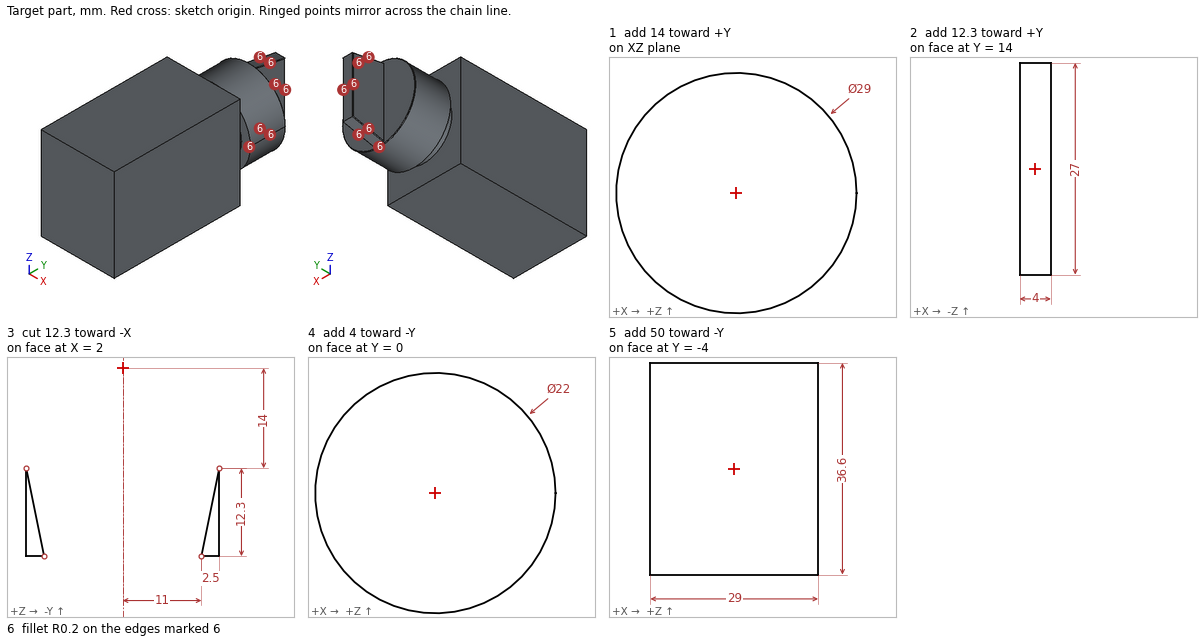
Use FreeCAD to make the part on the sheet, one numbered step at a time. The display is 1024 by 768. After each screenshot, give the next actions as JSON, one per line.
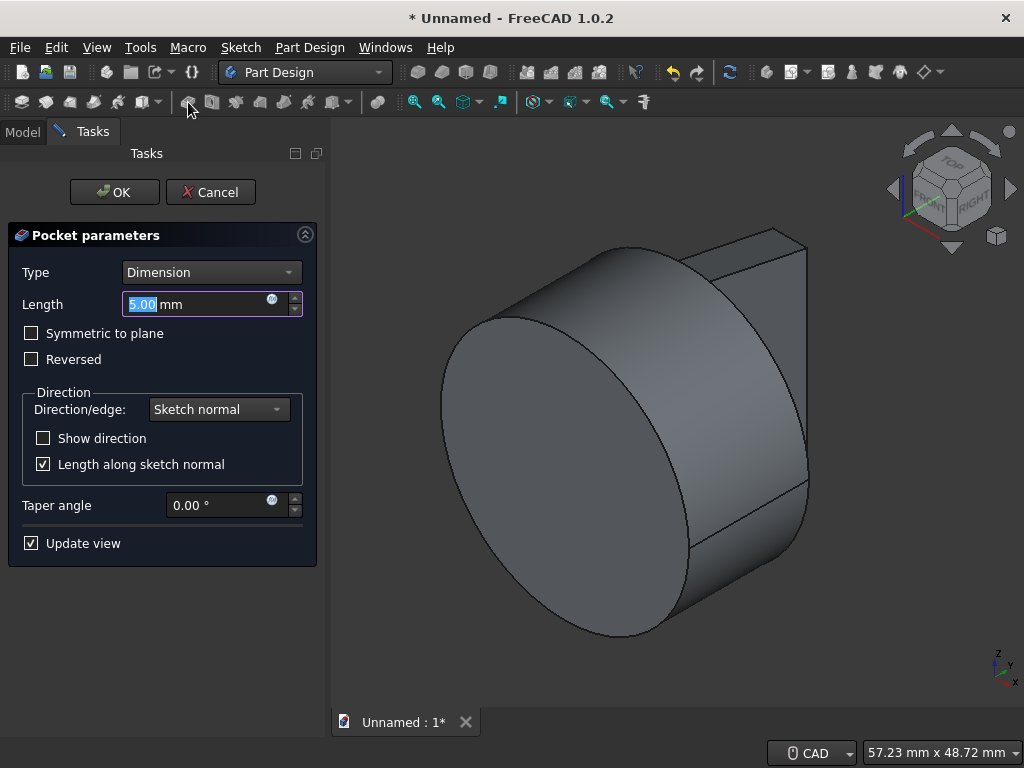
{"action": "type", "text": "12.3"}
{"action": "key", "text": "Tab"}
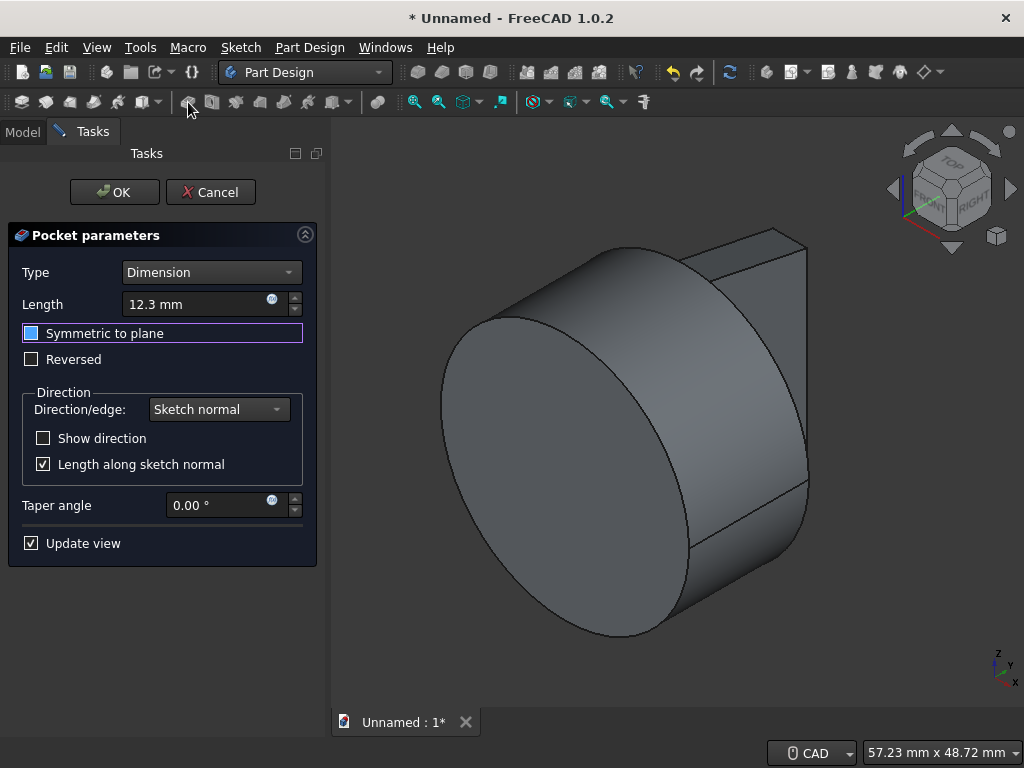
{"action": "left_click", "coordinate": [115, 192]}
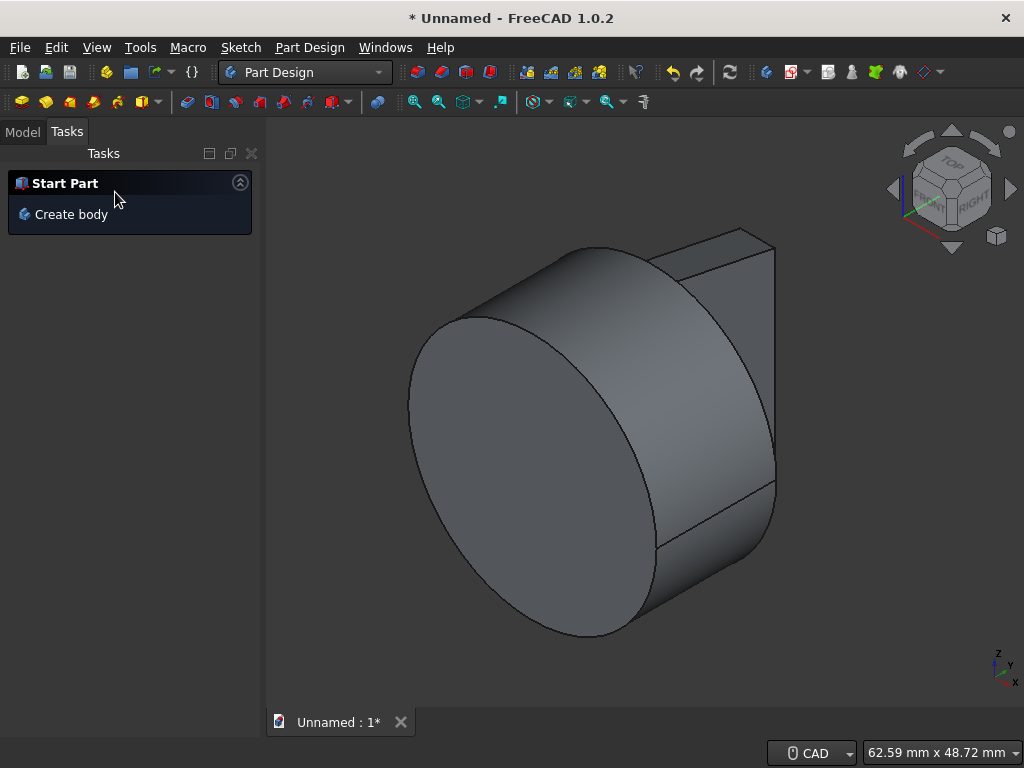
{"action": "left_click", "coordinate": [532, 476]}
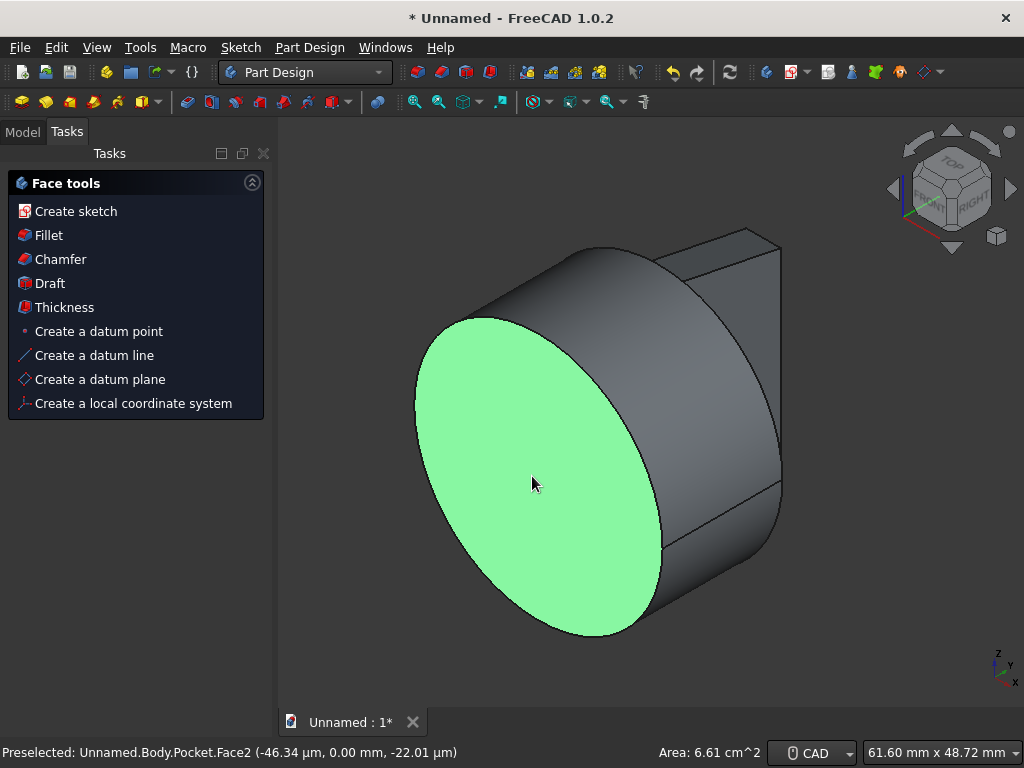
{"action": "left_click", "coordinate": [792, 72]}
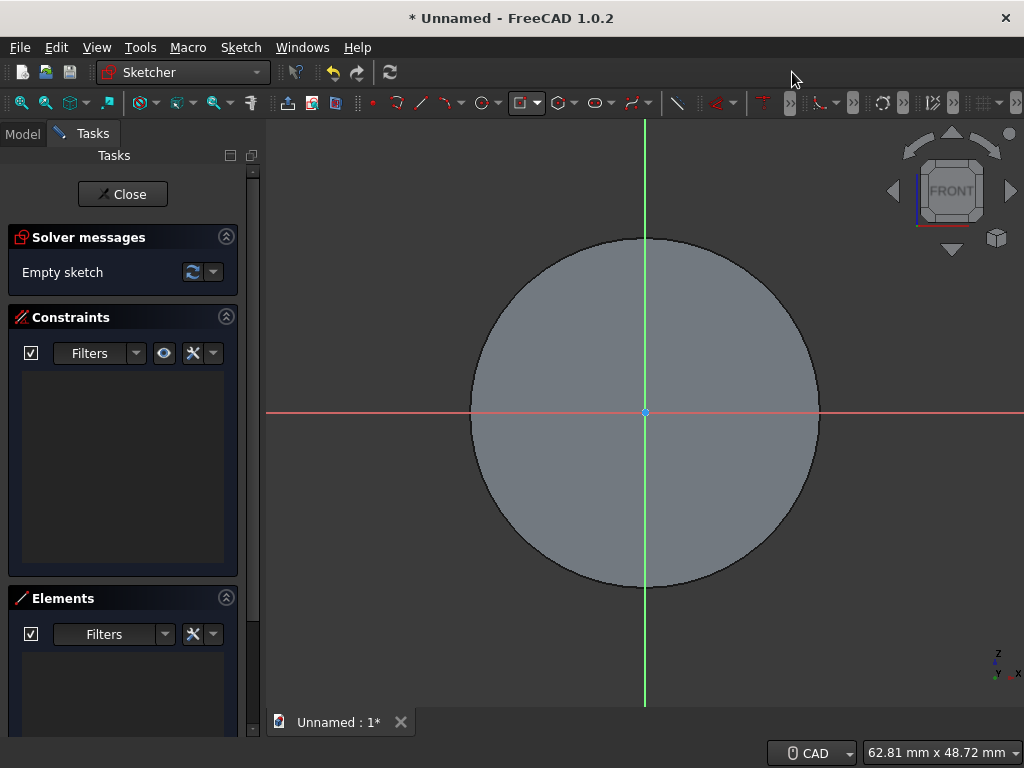
{"action": "scroll", "coordinate": [784, 413], "scroll_direction": "up", "scroll_amount": 2}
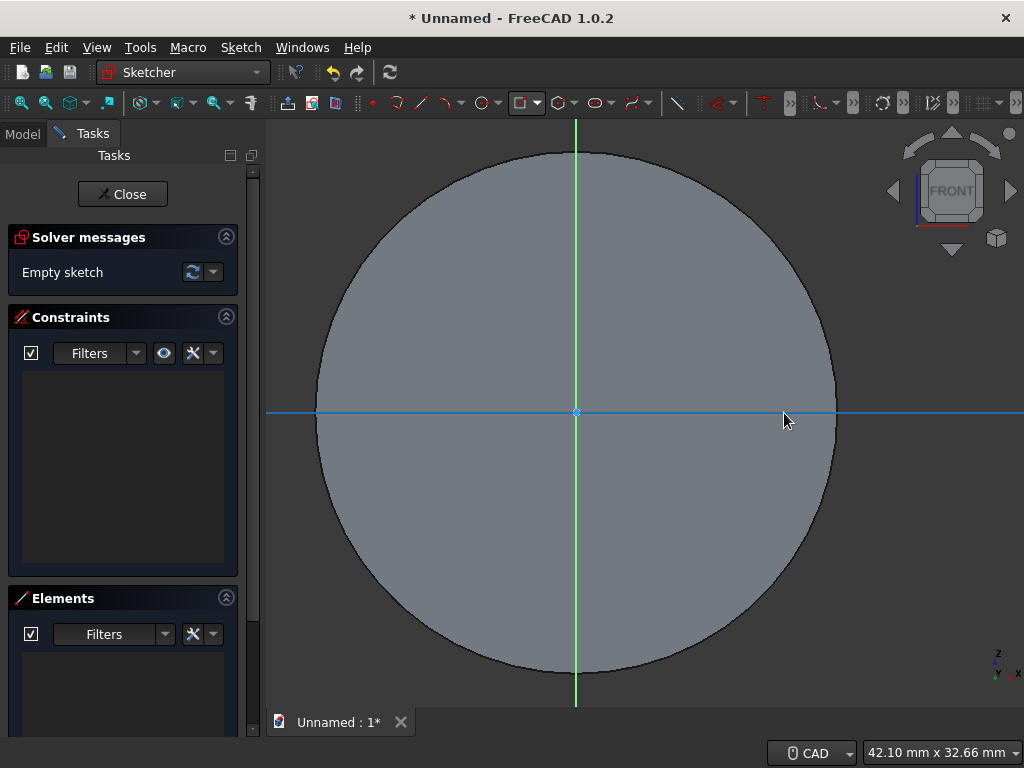
{"action": "left_click", "coordinate": [482, 104]}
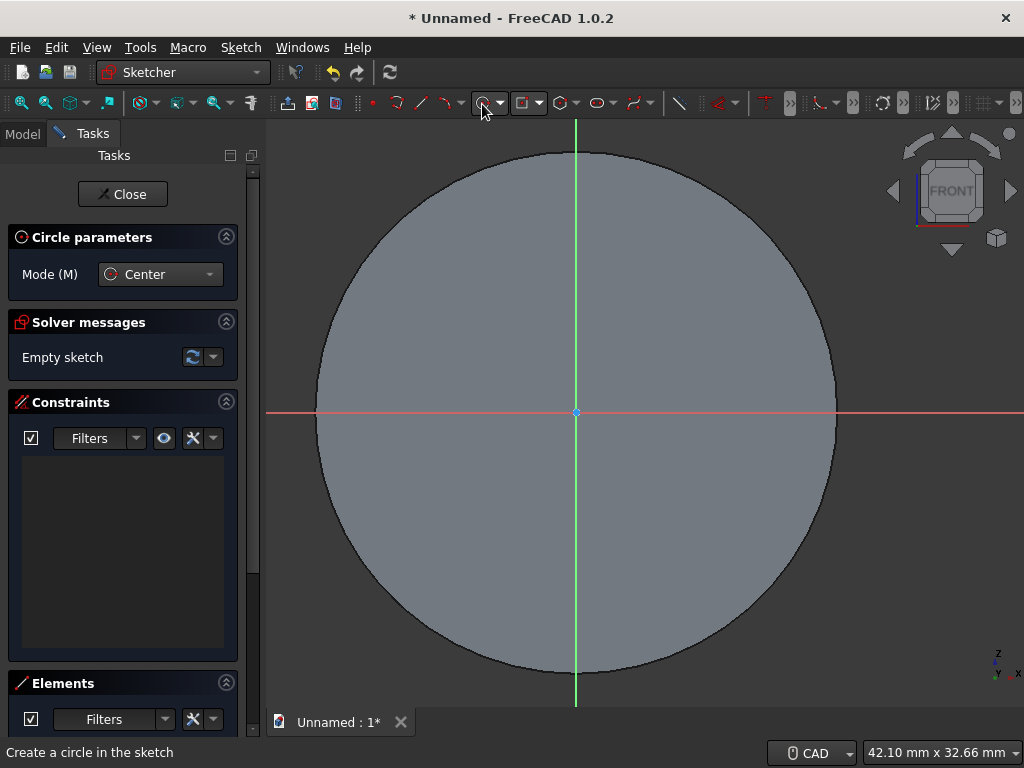
{"action": "left_click", "coordinate": [576, 413]}
{"action": "mouse_move", "coordinate": [716, 273]}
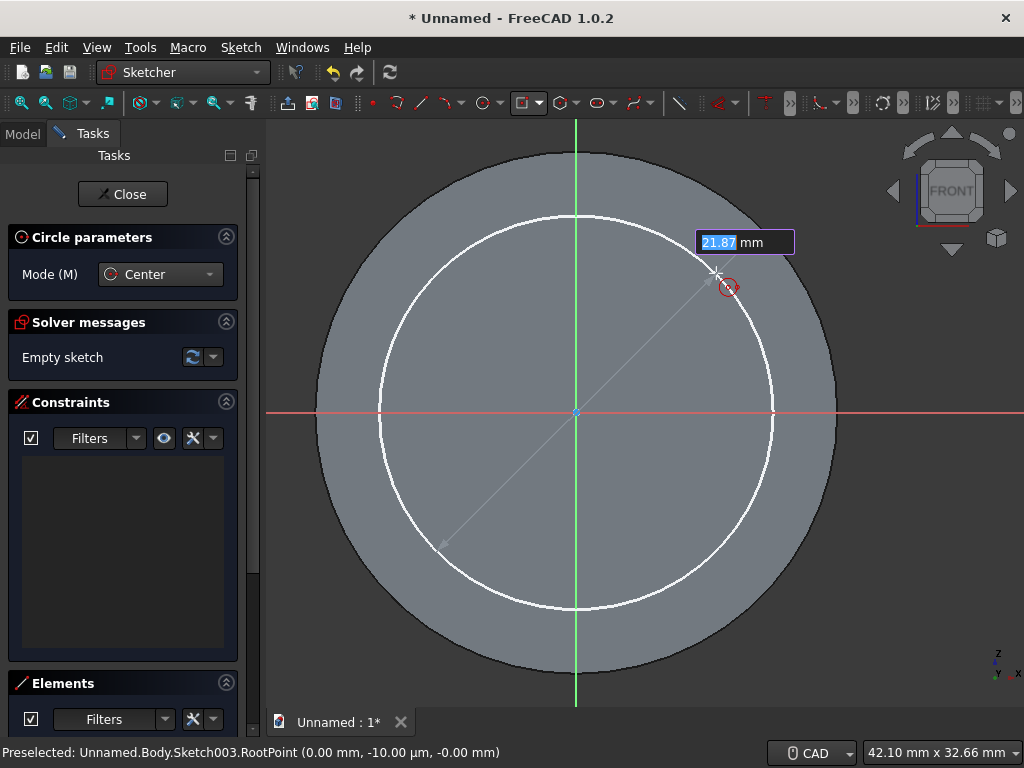
{"action": "type", "text": "22"}
{"action": "key", "text": "Return"}
{"action": "key", "text": "Escape"}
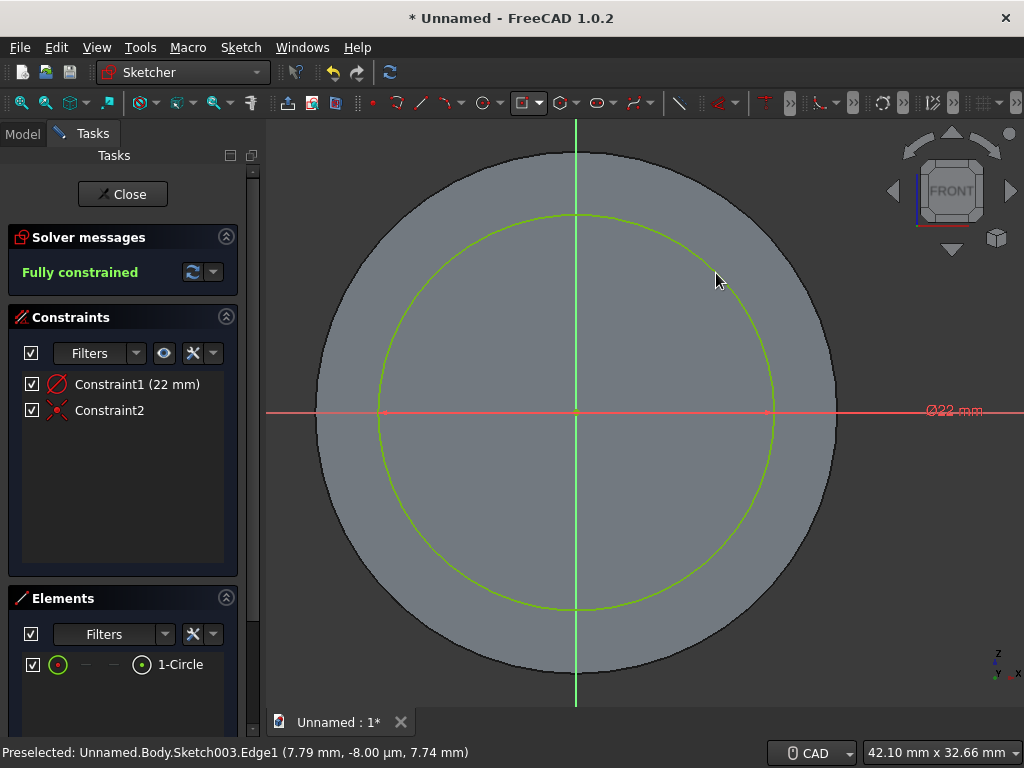
{"action": "left_click", "coordinate": [123, 194]}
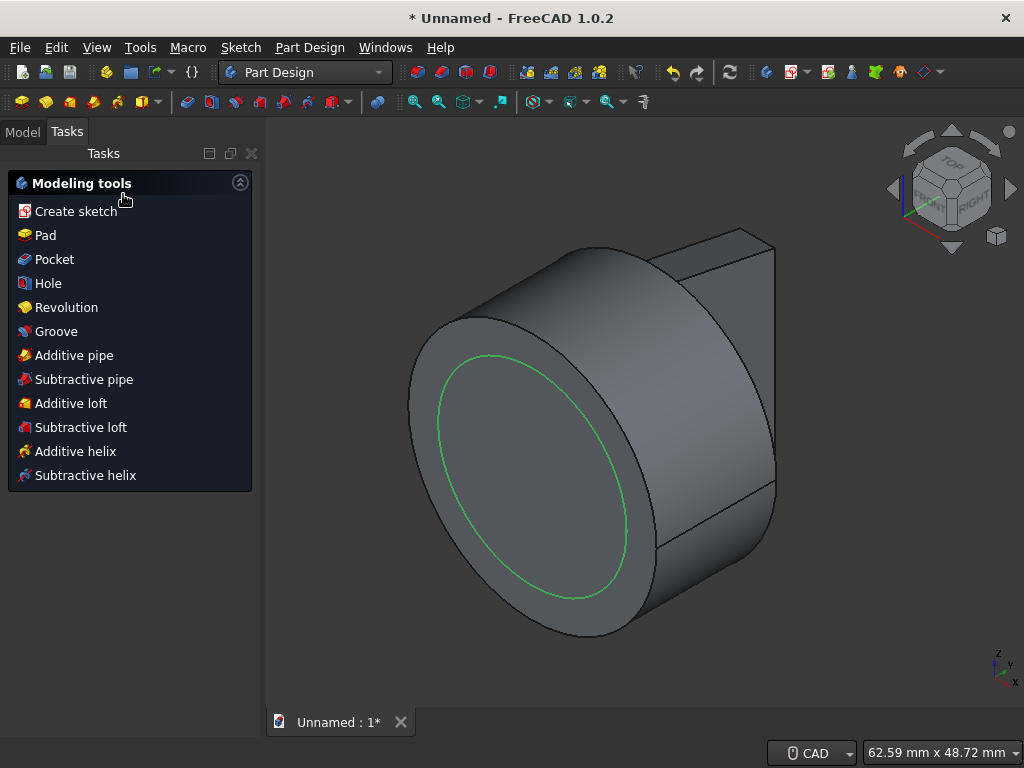
{"action": "left_click", "coordinate": [22, 102]}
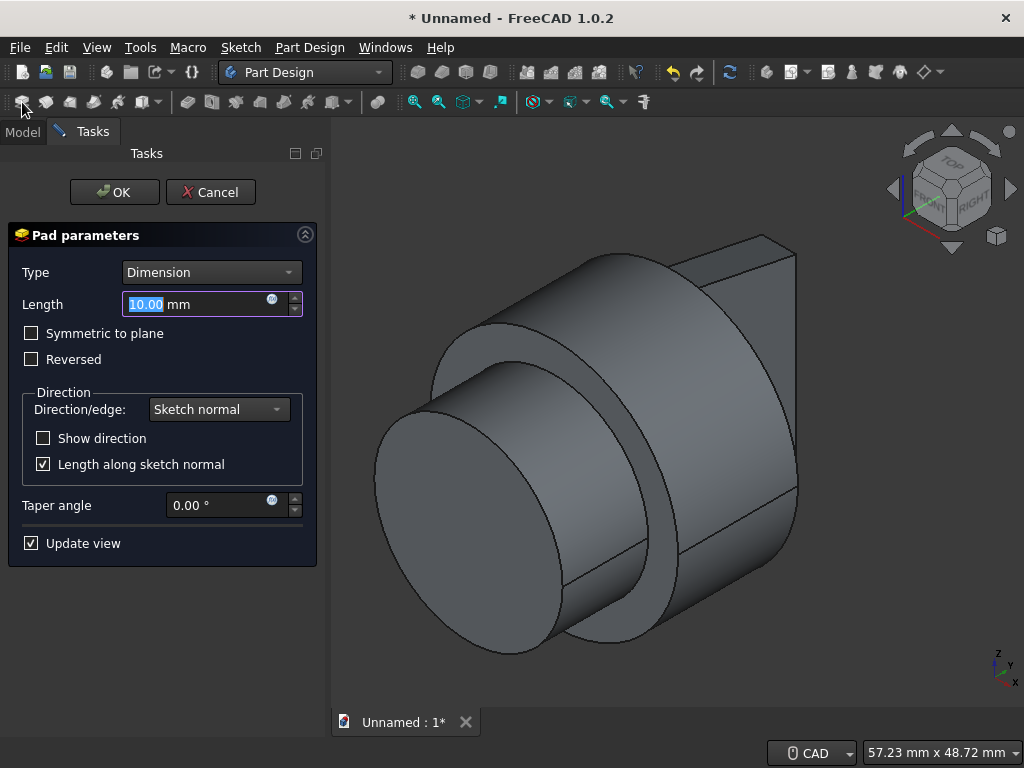
{"action": "type", "text": "4"}
{"action": "key", "text": "Tab"}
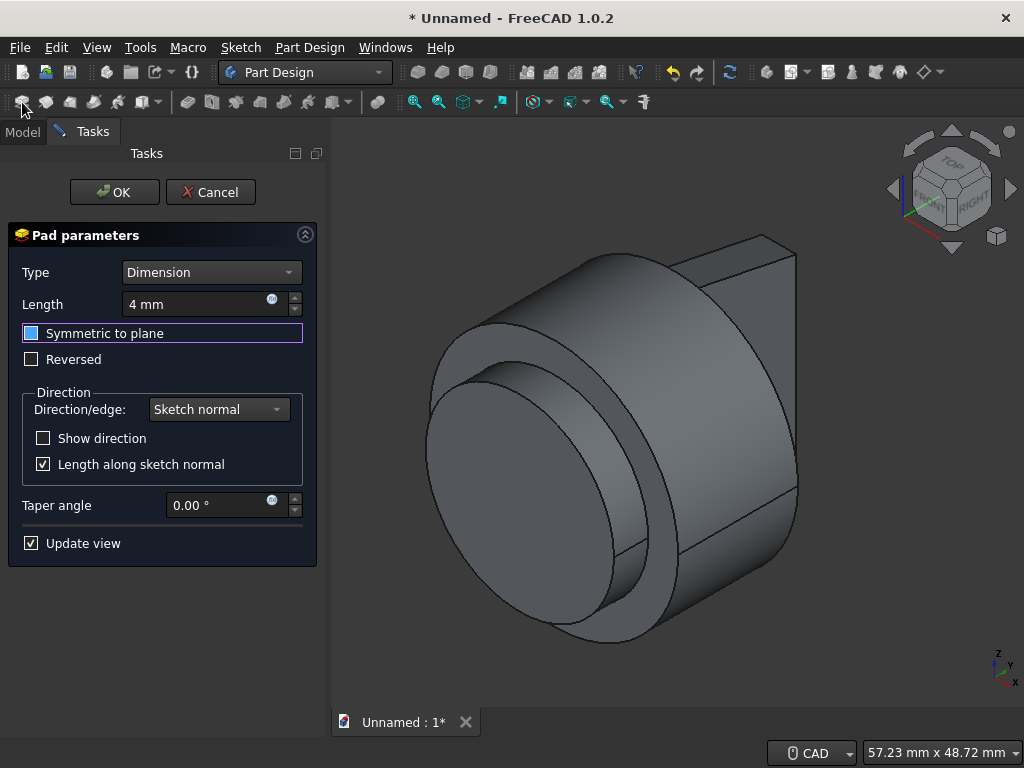
{"action": "left_click", "coordinate": [115, 192]}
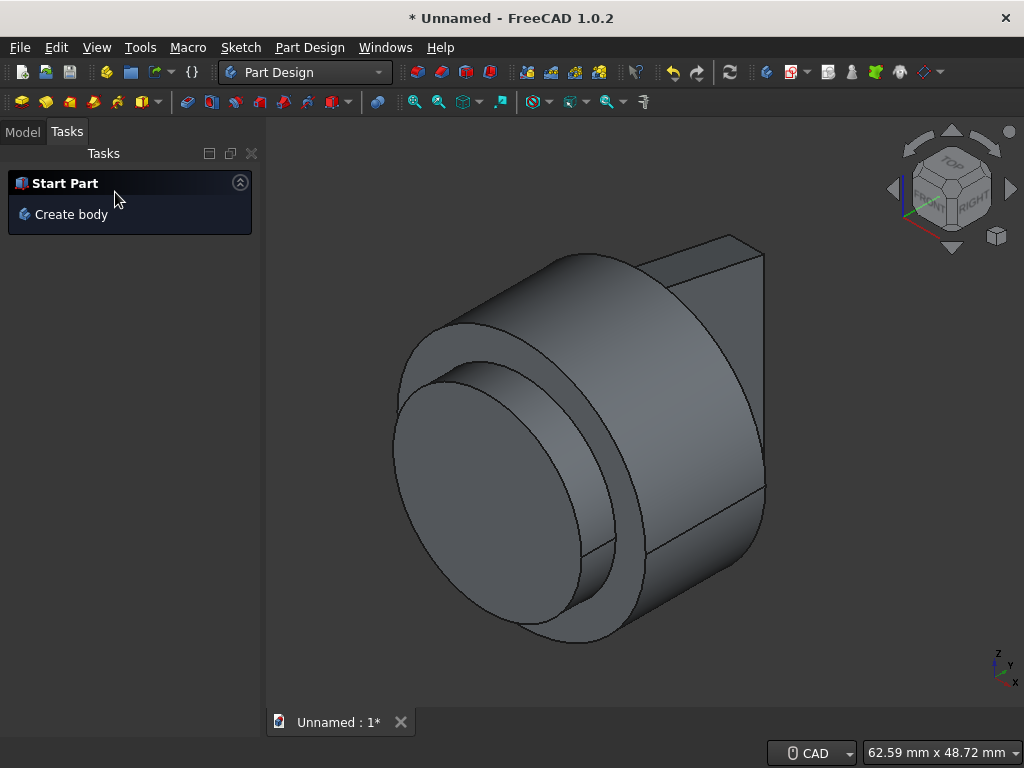
{"action": "left_click", "coordinate": [416, 102]}